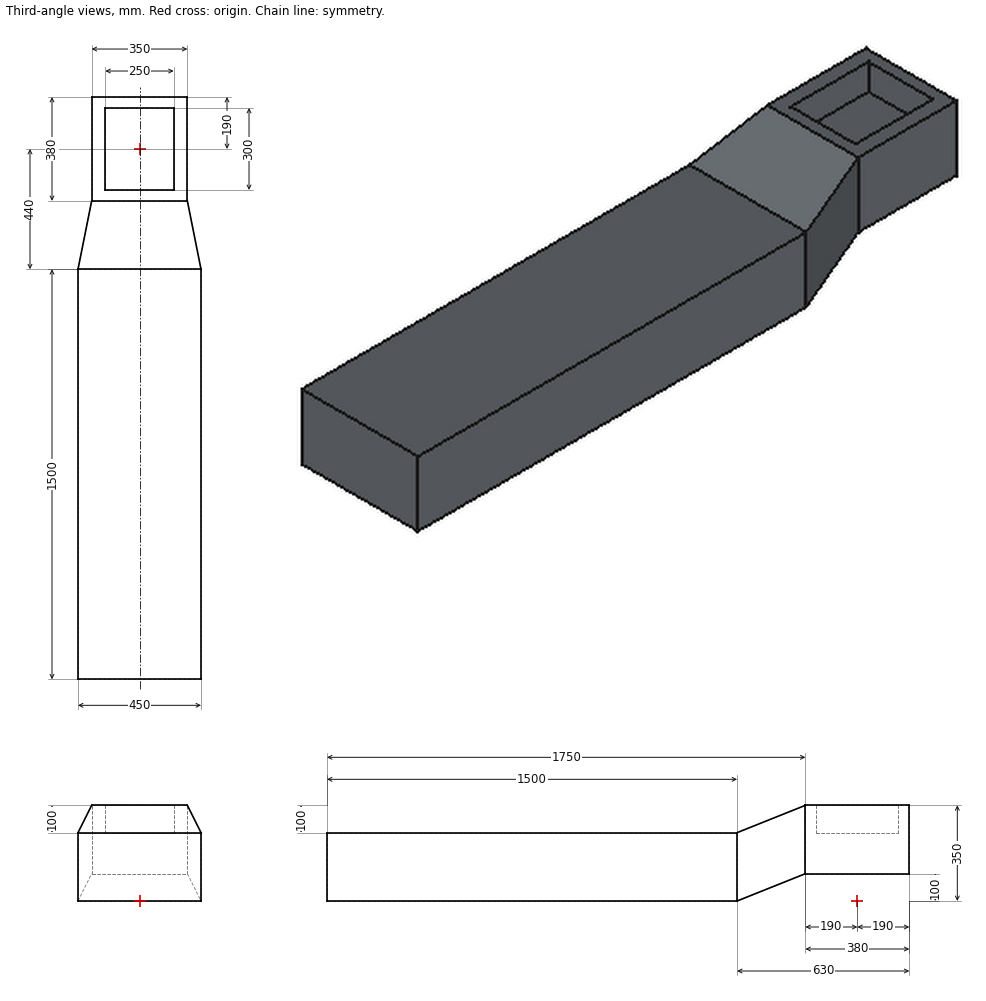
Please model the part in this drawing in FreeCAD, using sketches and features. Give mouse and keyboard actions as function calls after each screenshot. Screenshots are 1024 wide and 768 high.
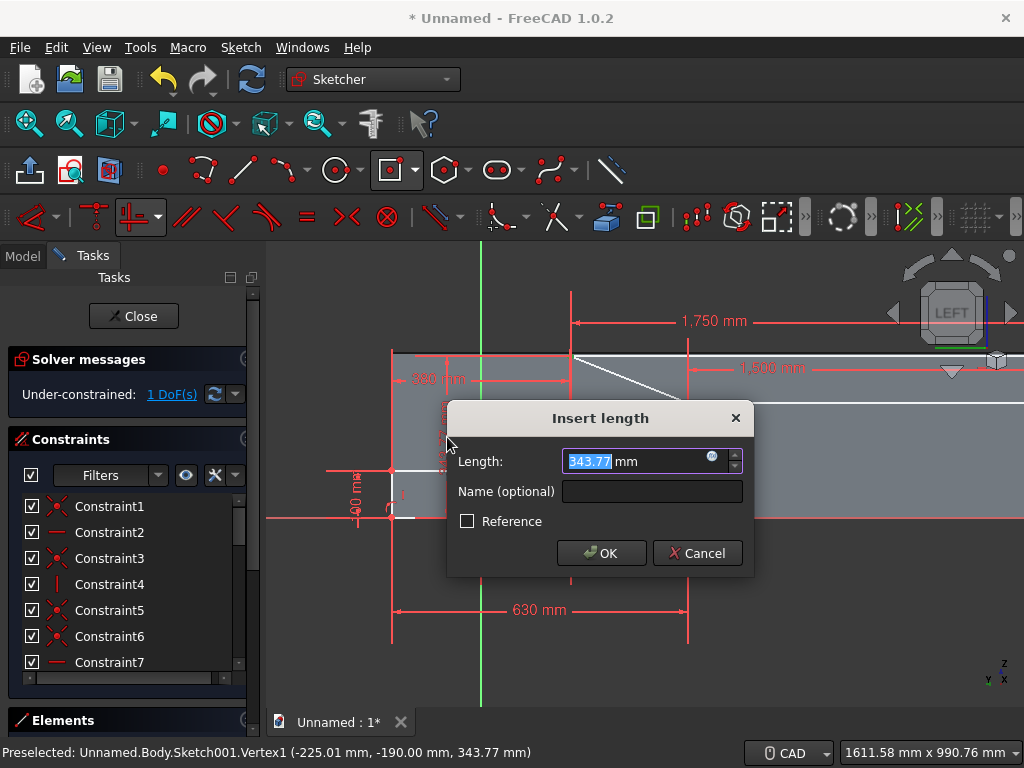
text(350)
key(Return)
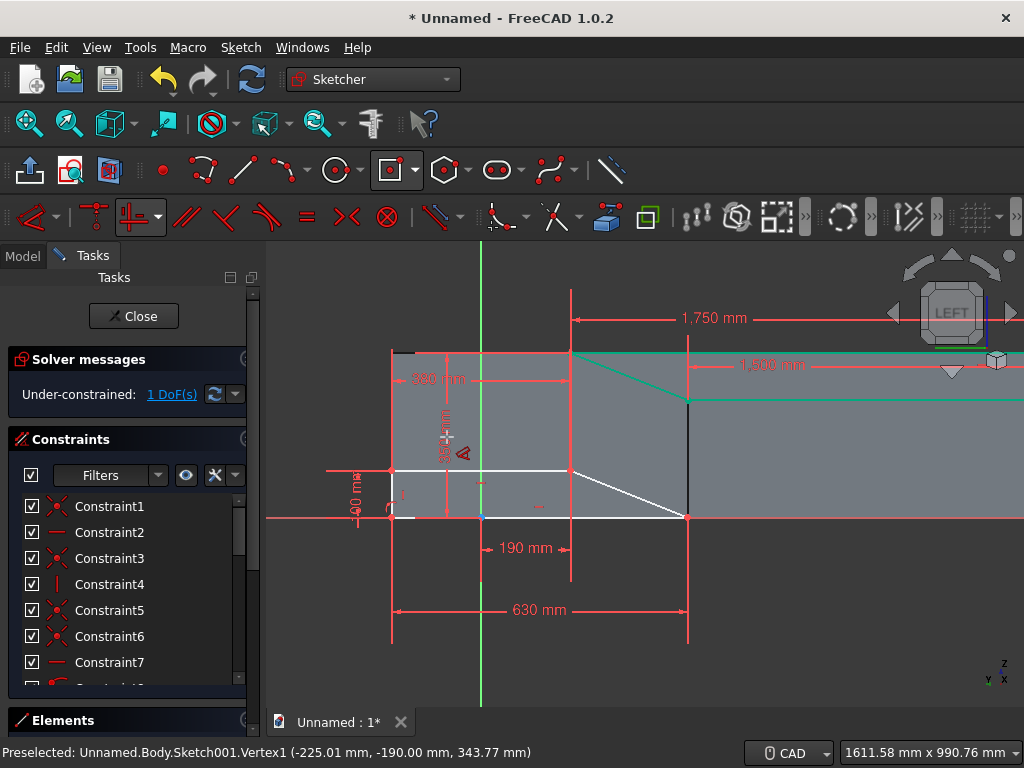
click(392, 518)
click(436, 552)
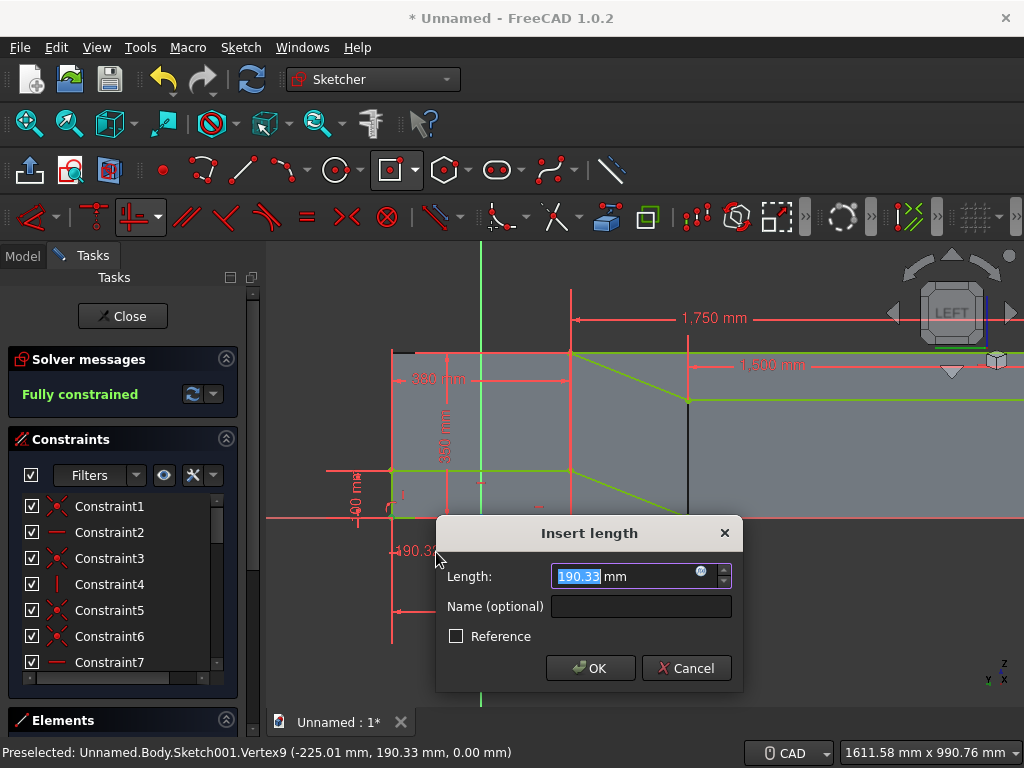
text(190)
key(Return)
key(Escape)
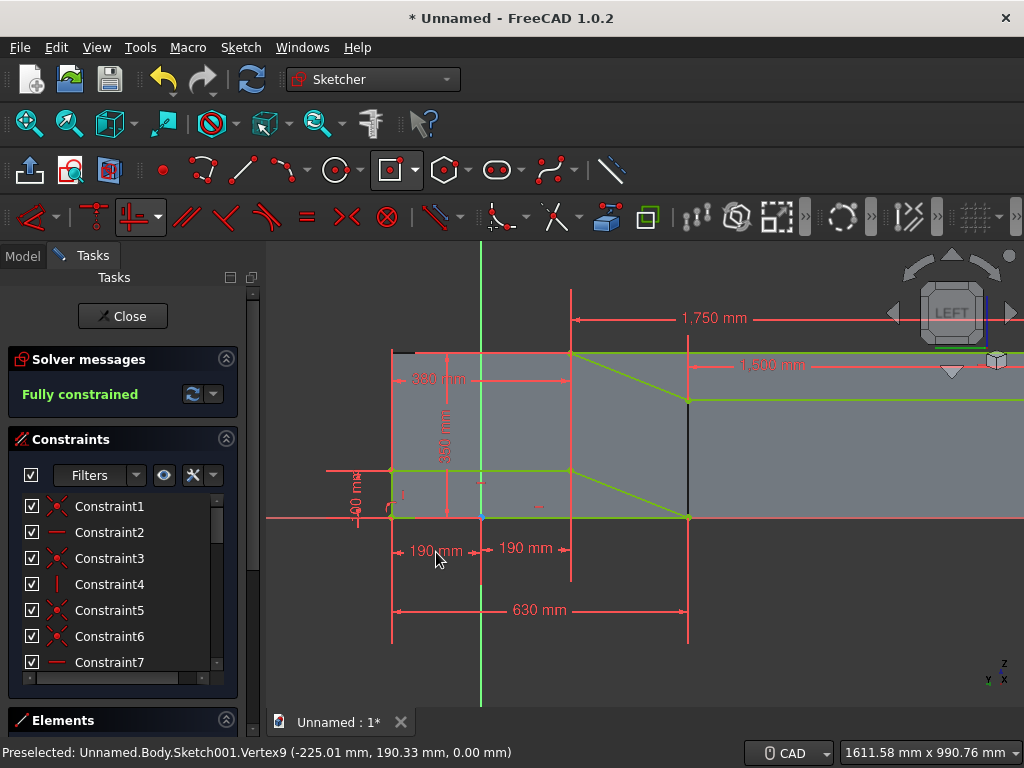
click(123, 316)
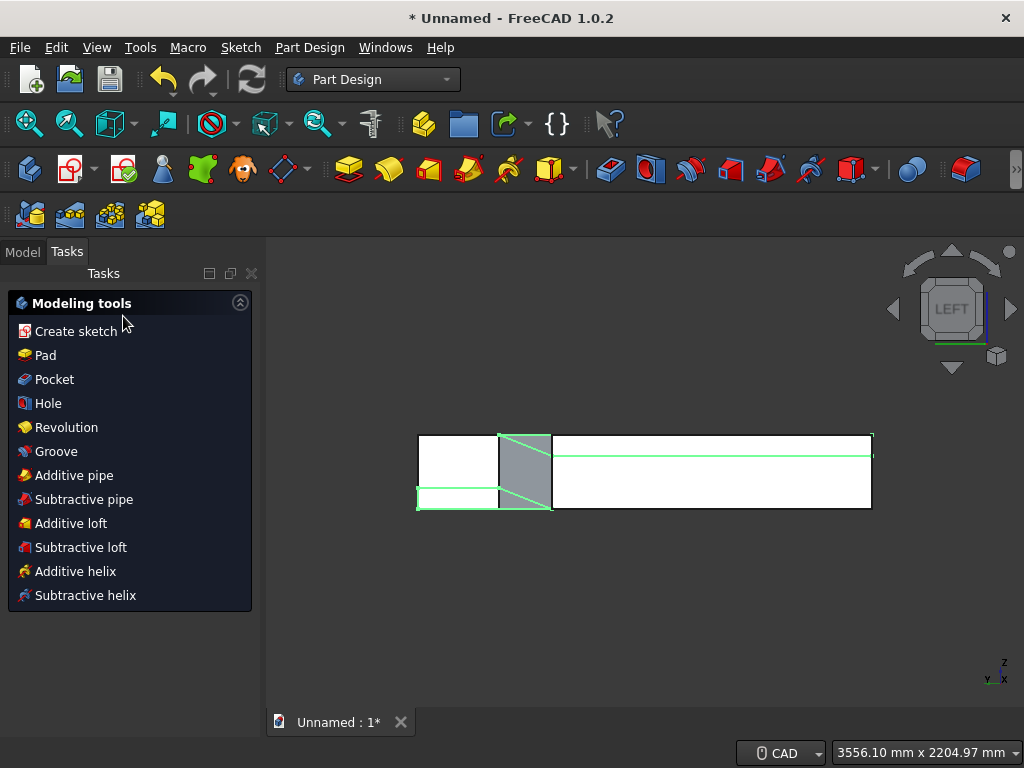
click(612, 170)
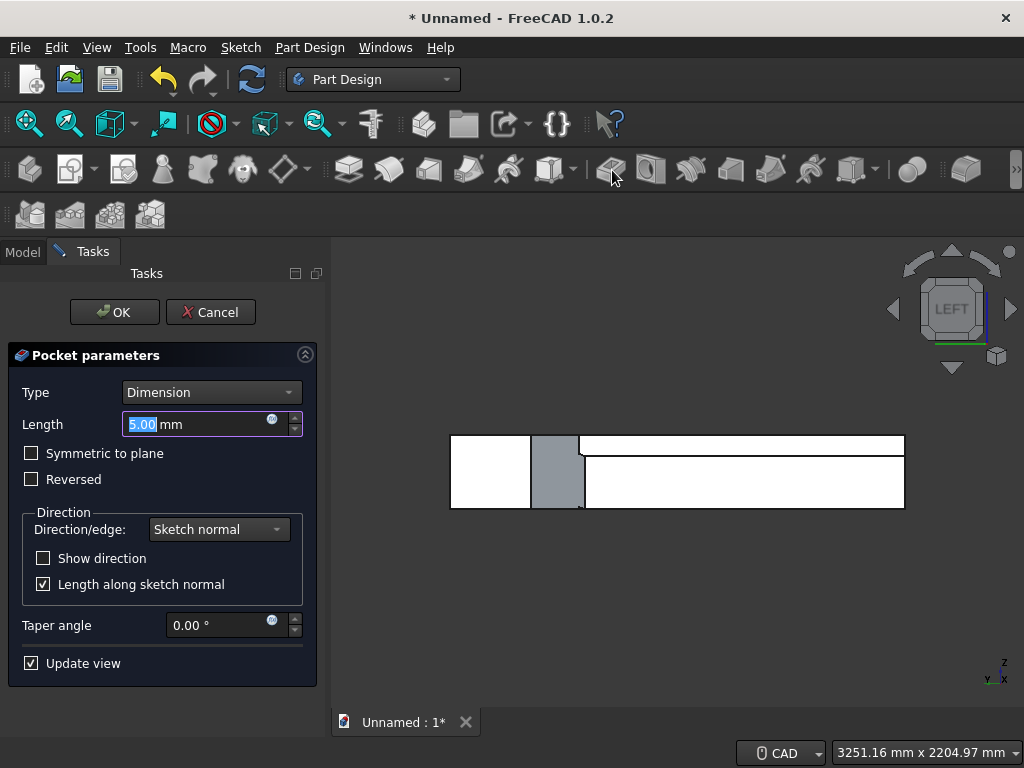
click(212, 392)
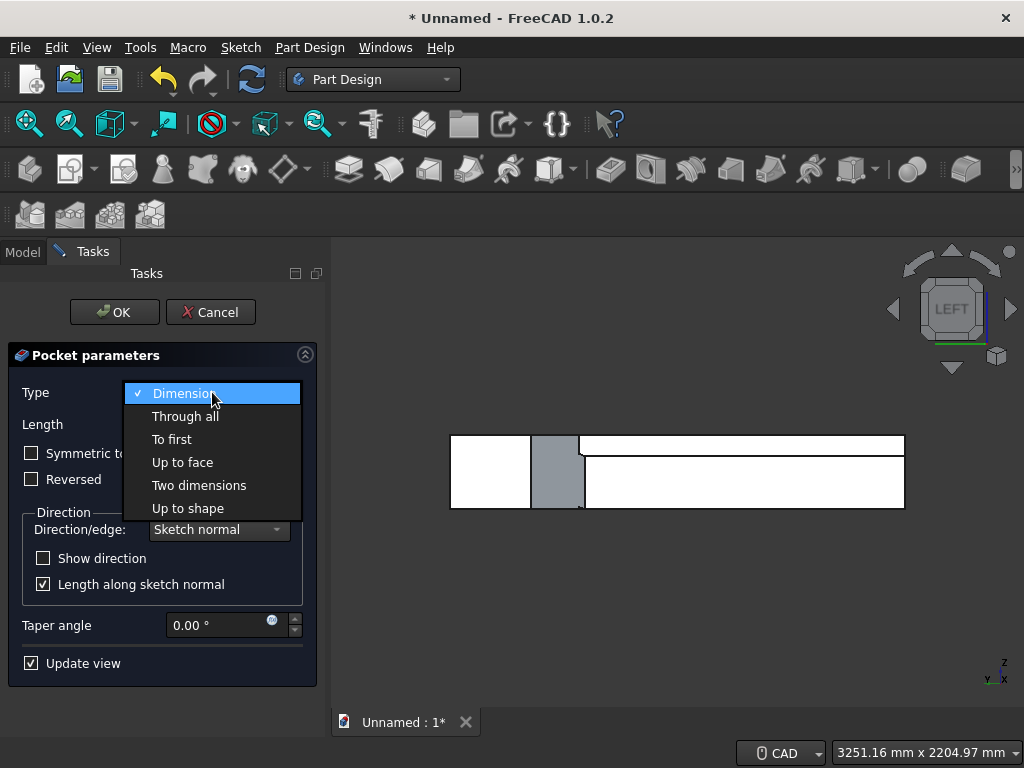
click(212, 416)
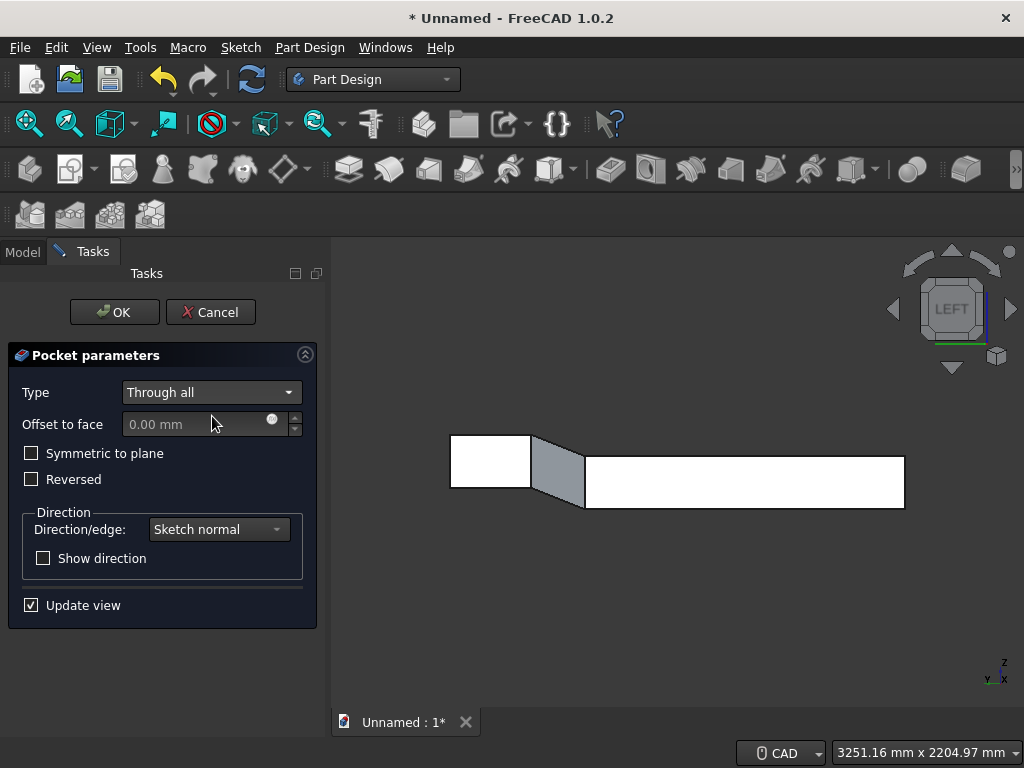
click(115, 312)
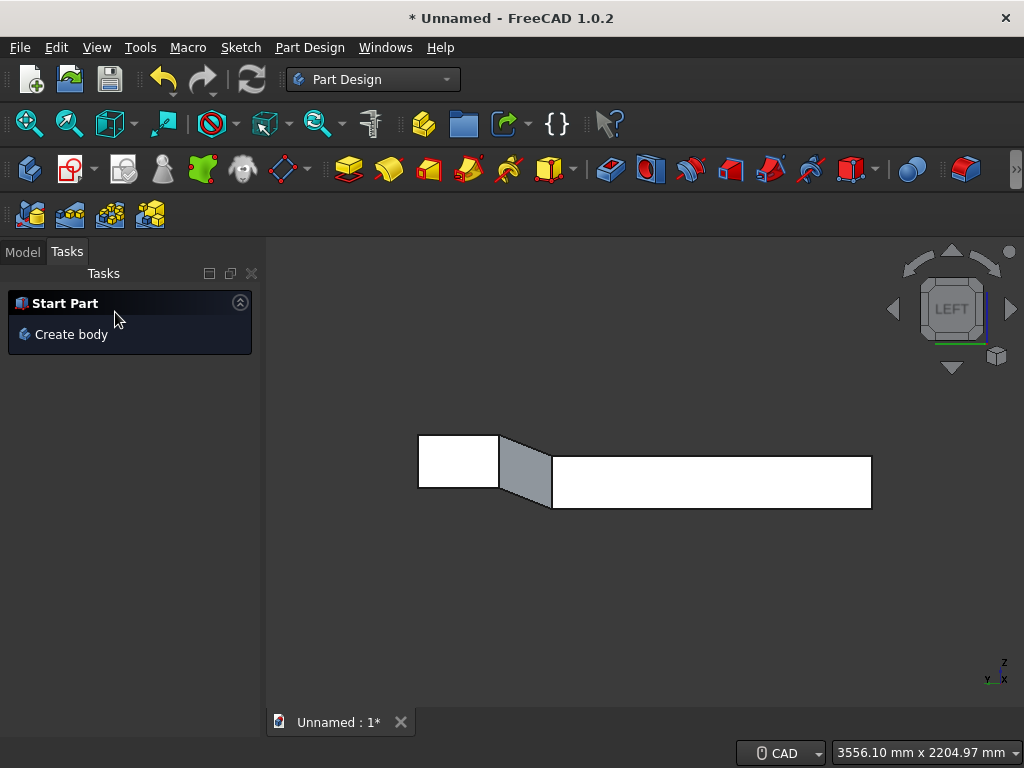
key(0)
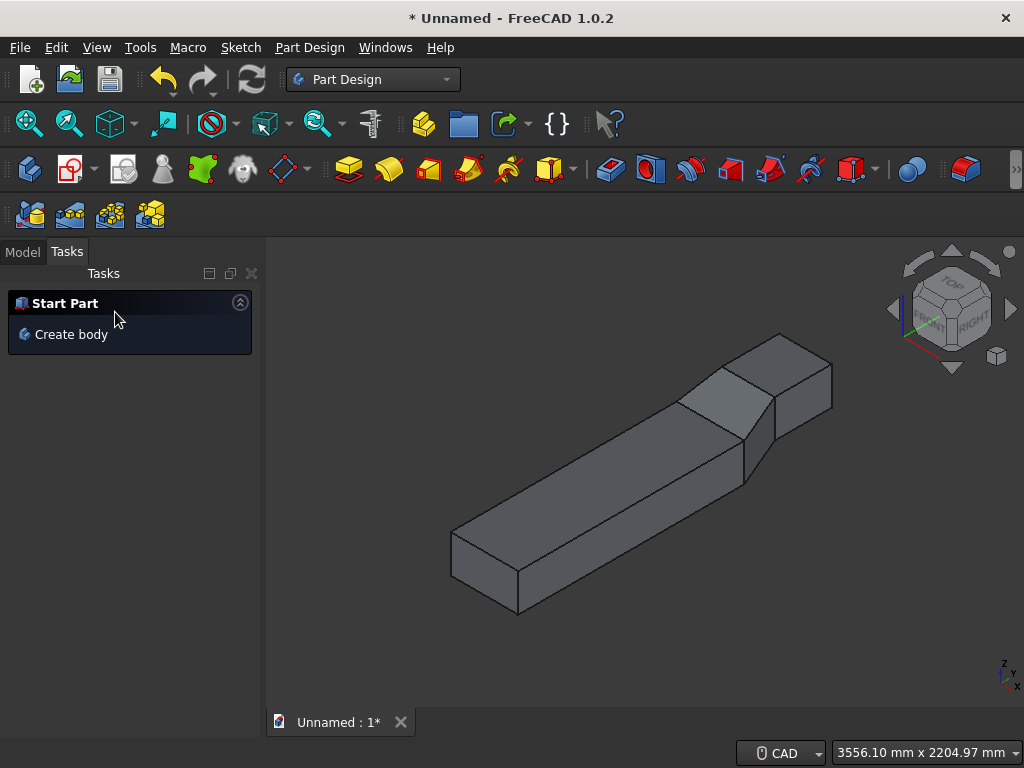
click(777, 364)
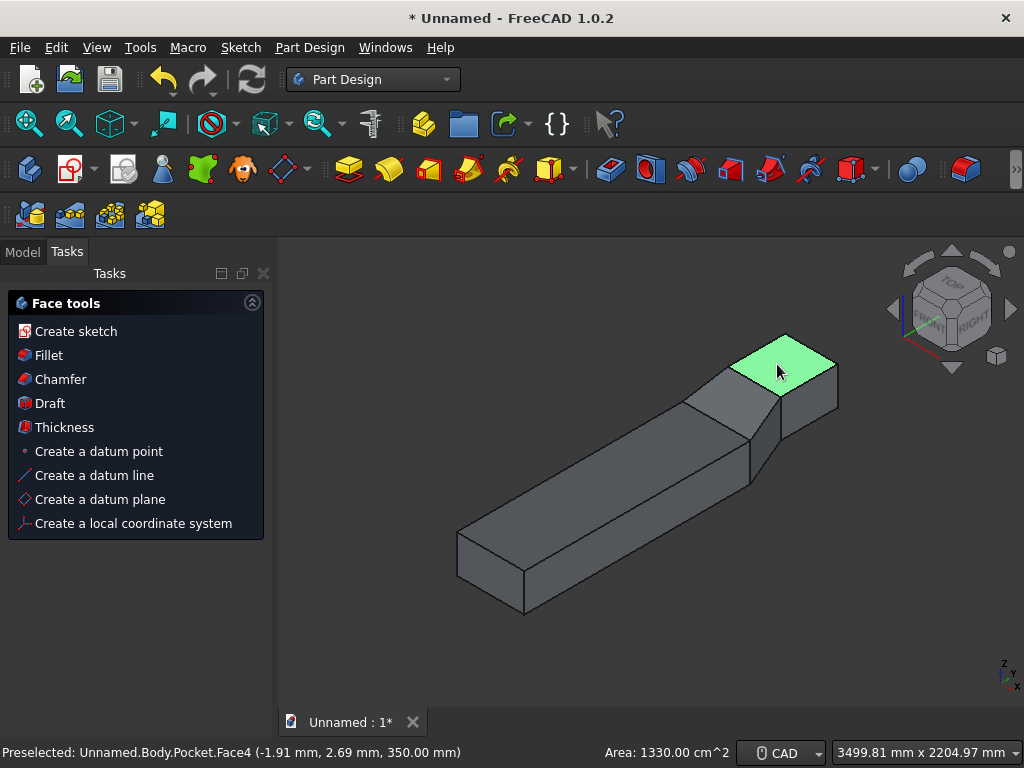
click(70, 170)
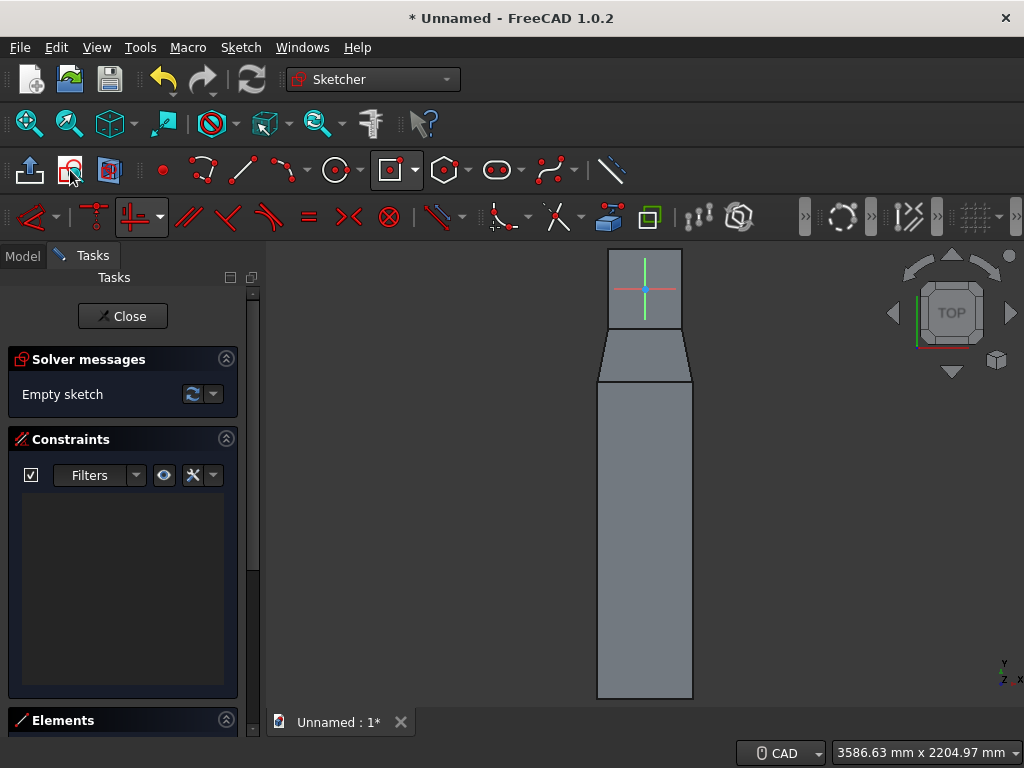
scroll(576, 474, down, 5)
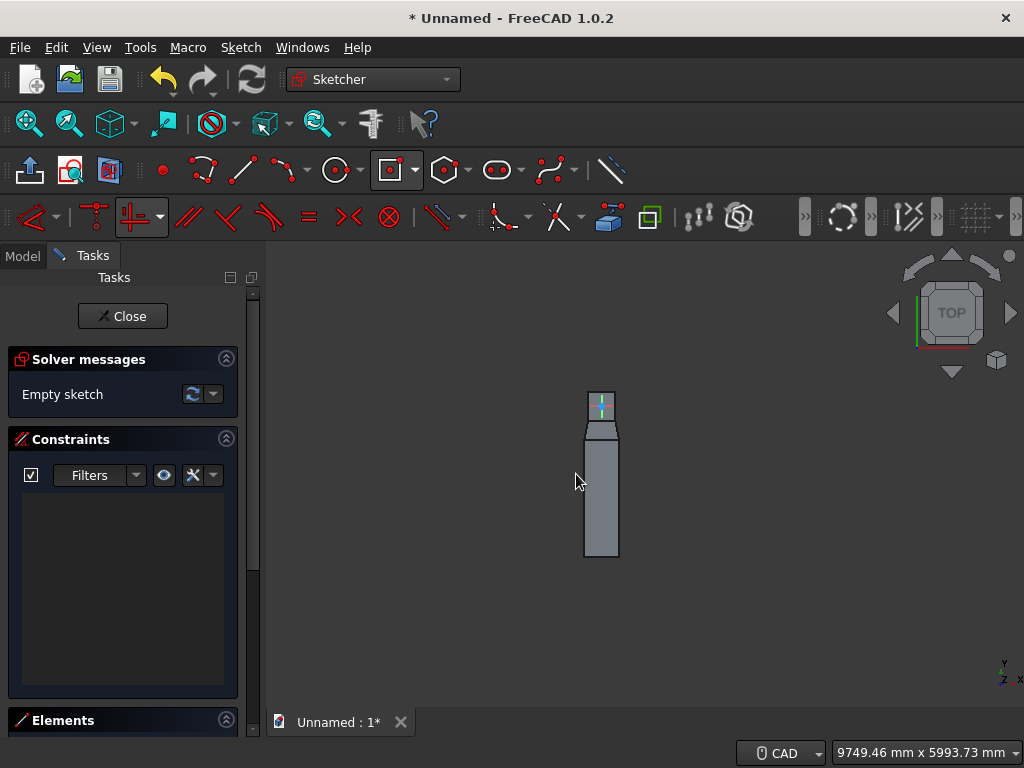
scroll(604, 401, up, 13)